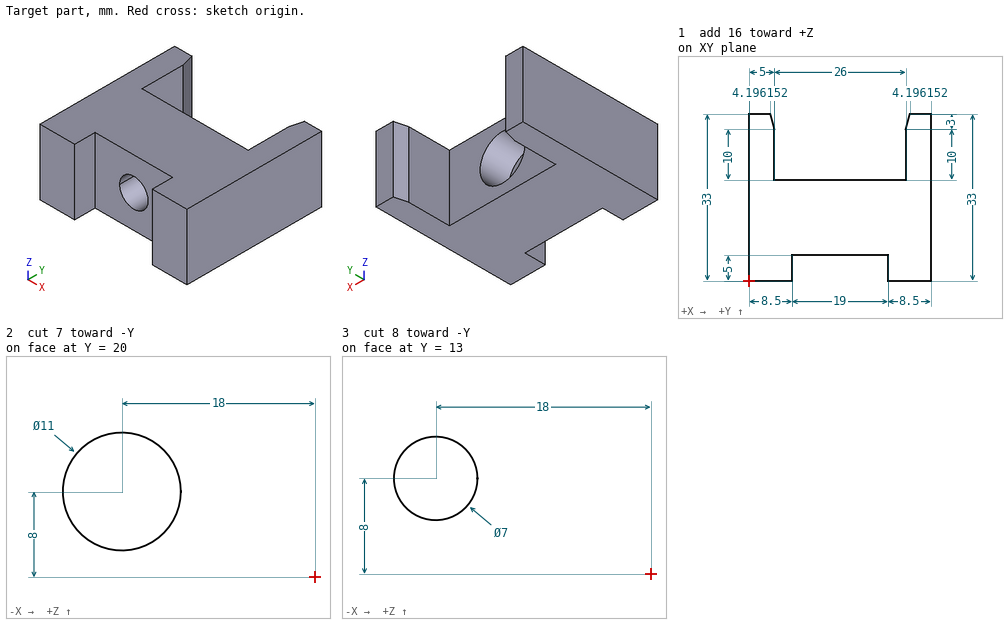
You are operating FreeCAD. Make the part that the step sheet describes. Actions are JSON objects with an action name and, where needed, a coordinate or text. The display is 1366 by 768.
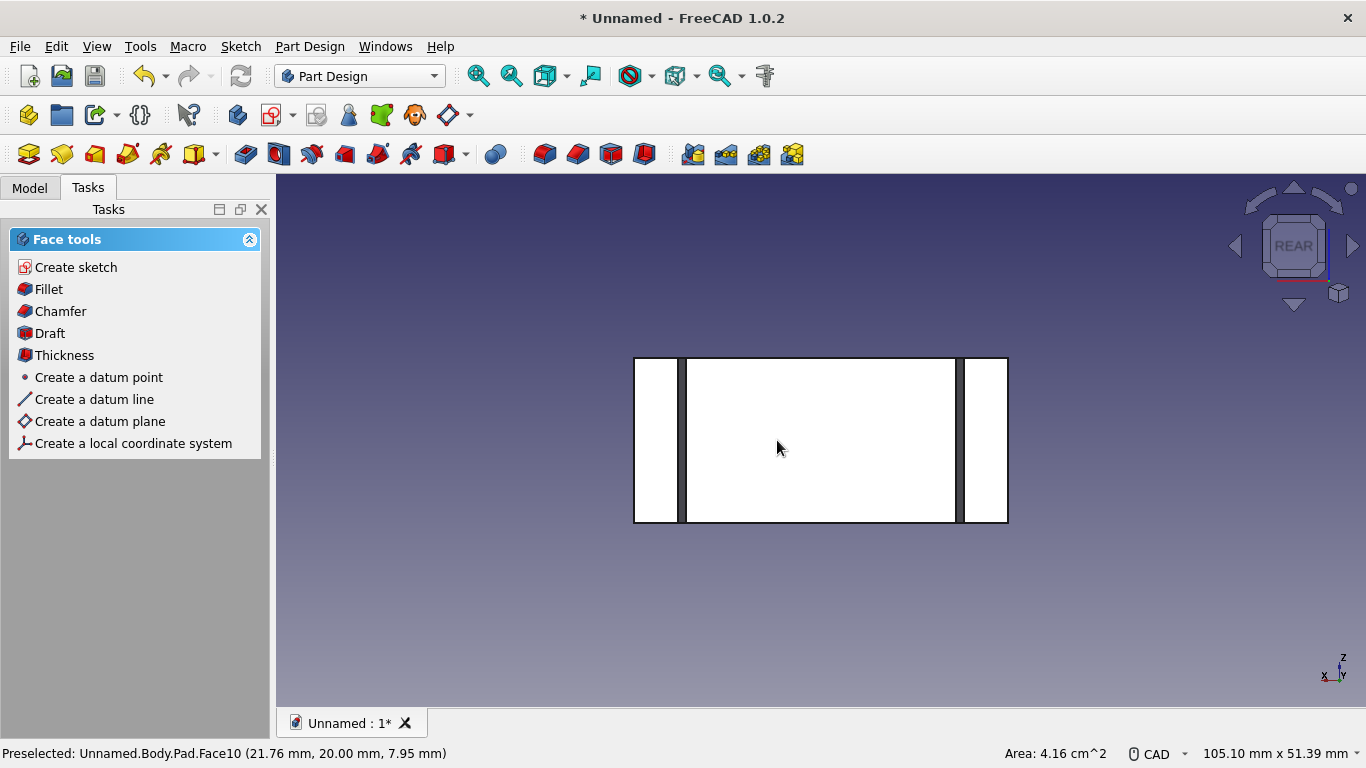
{"action": "left_click", "coordinate": [270, 116]}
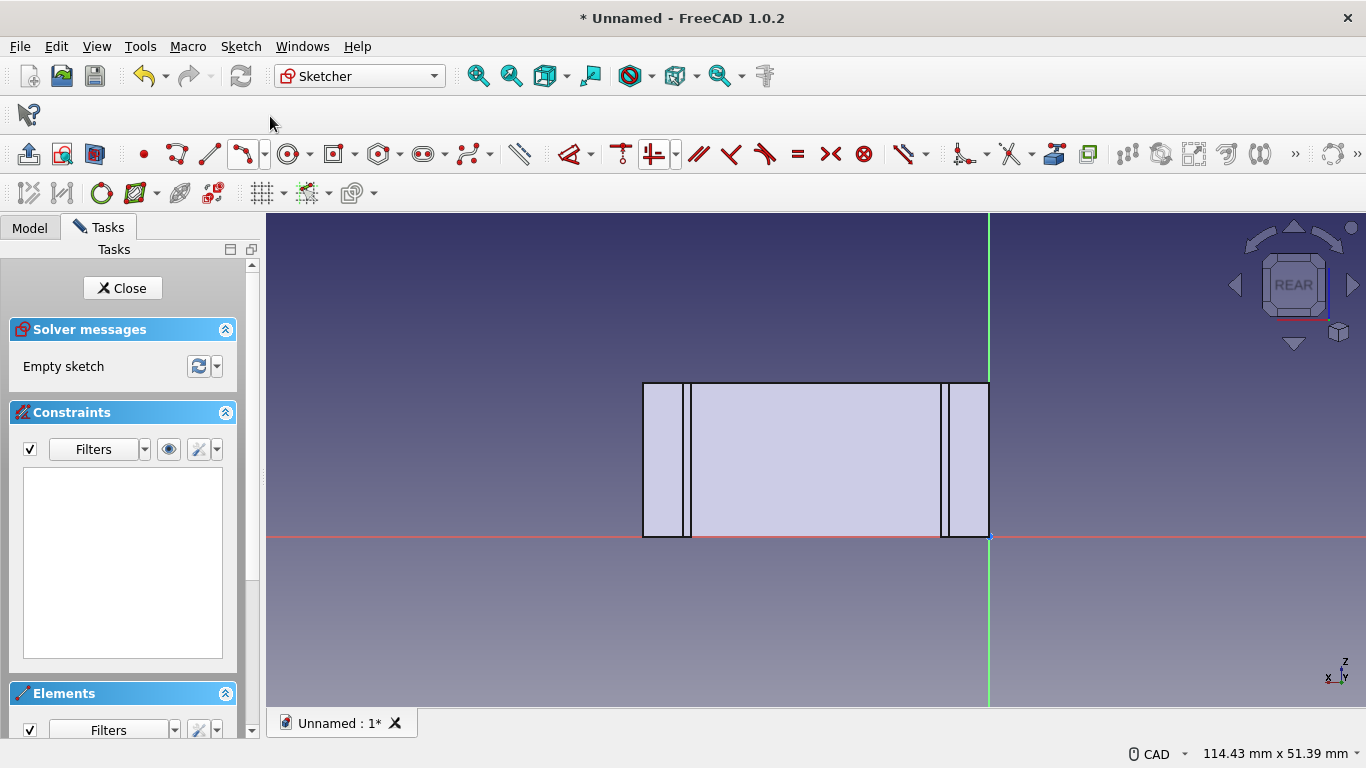
{"action": "left_click", "coordinate": [95, 154]}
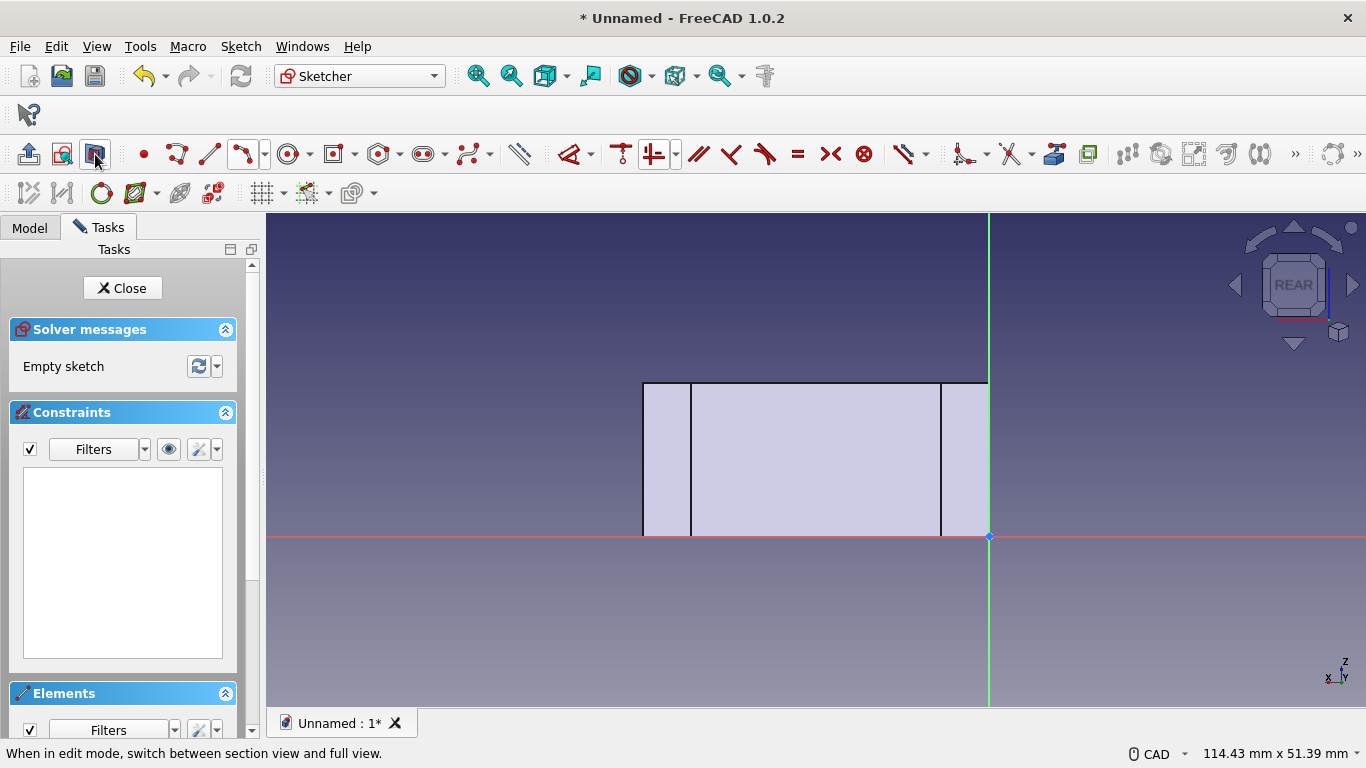
{"action": "scroll", "coordinate": [981, 482], "scroll_direction": "up", "scroll_amount": 4}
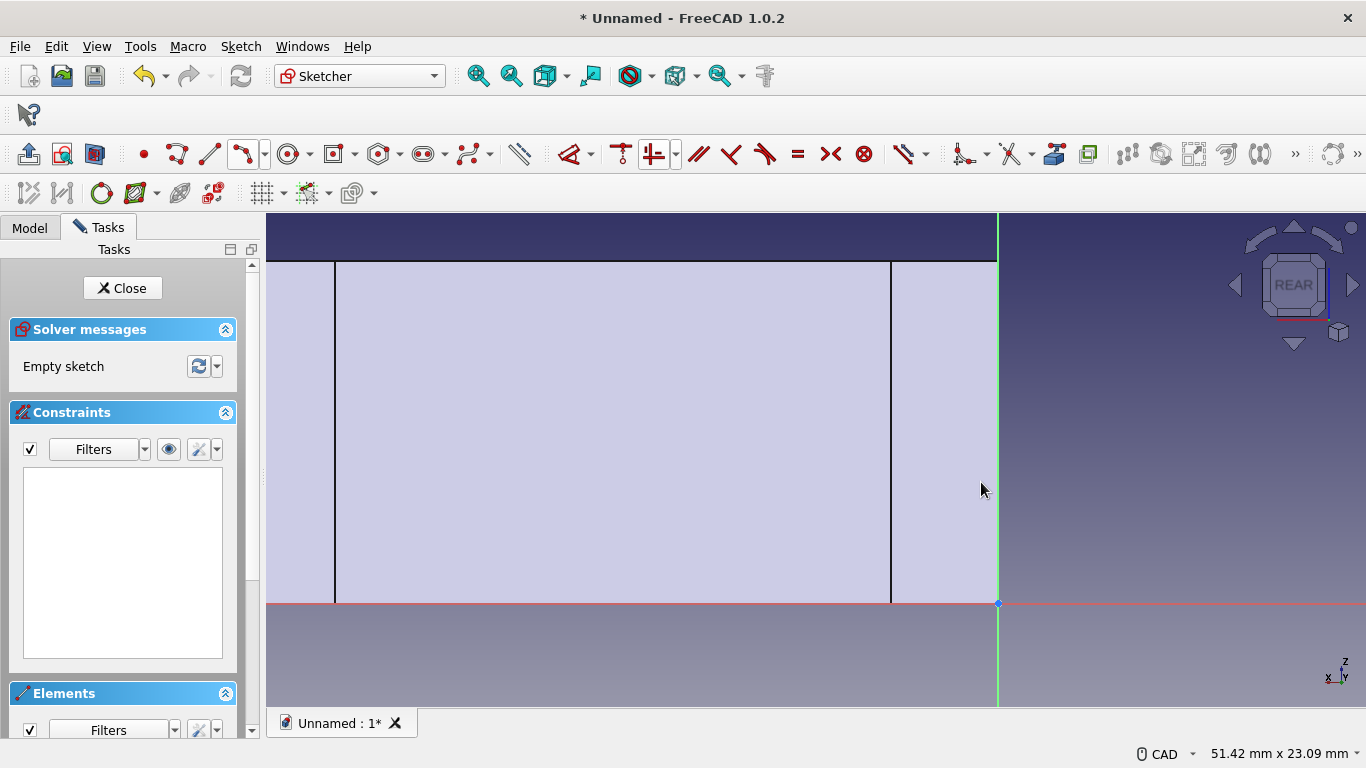
{"action": "left_click", "coordinate": [288, 154]}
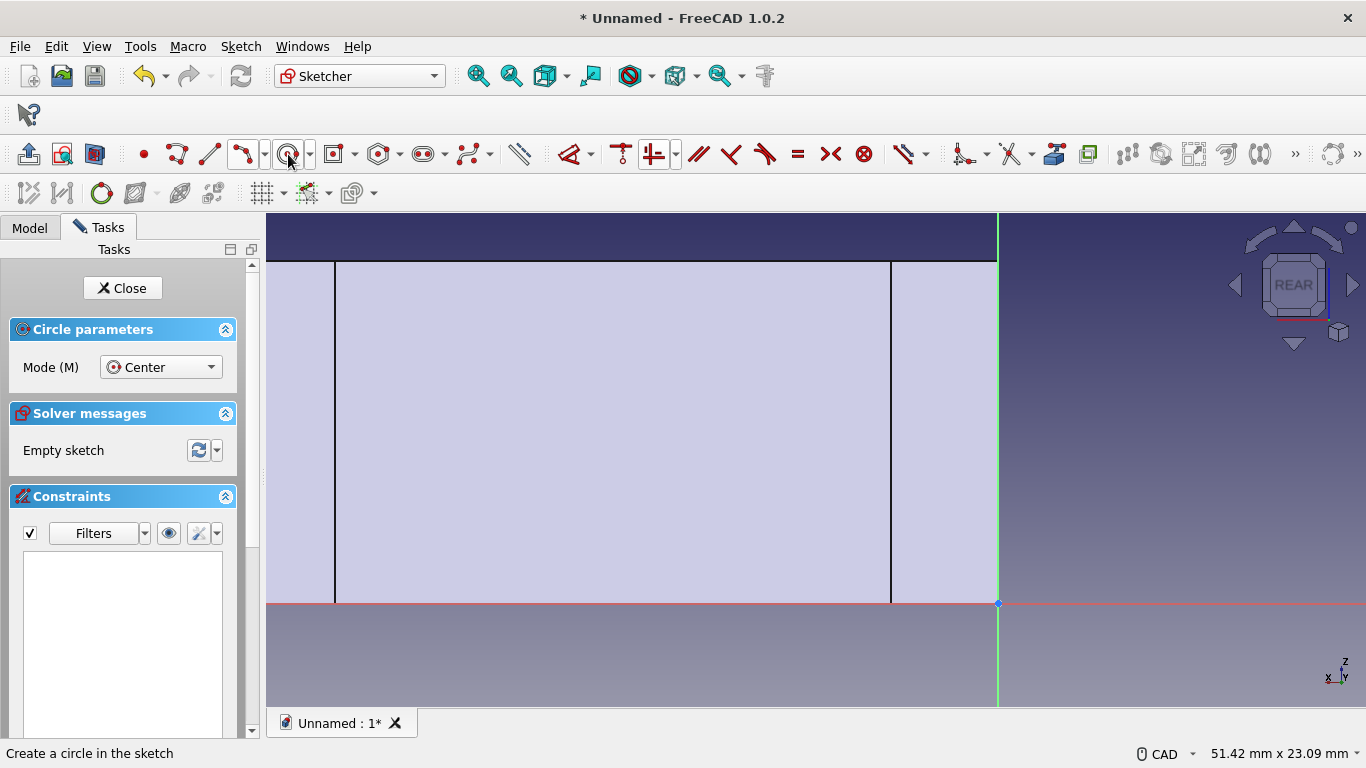
{"action": "left_click", "coordinate": [613, 432]}
{"action": "mouse_move", "coordinate": [696, 349]}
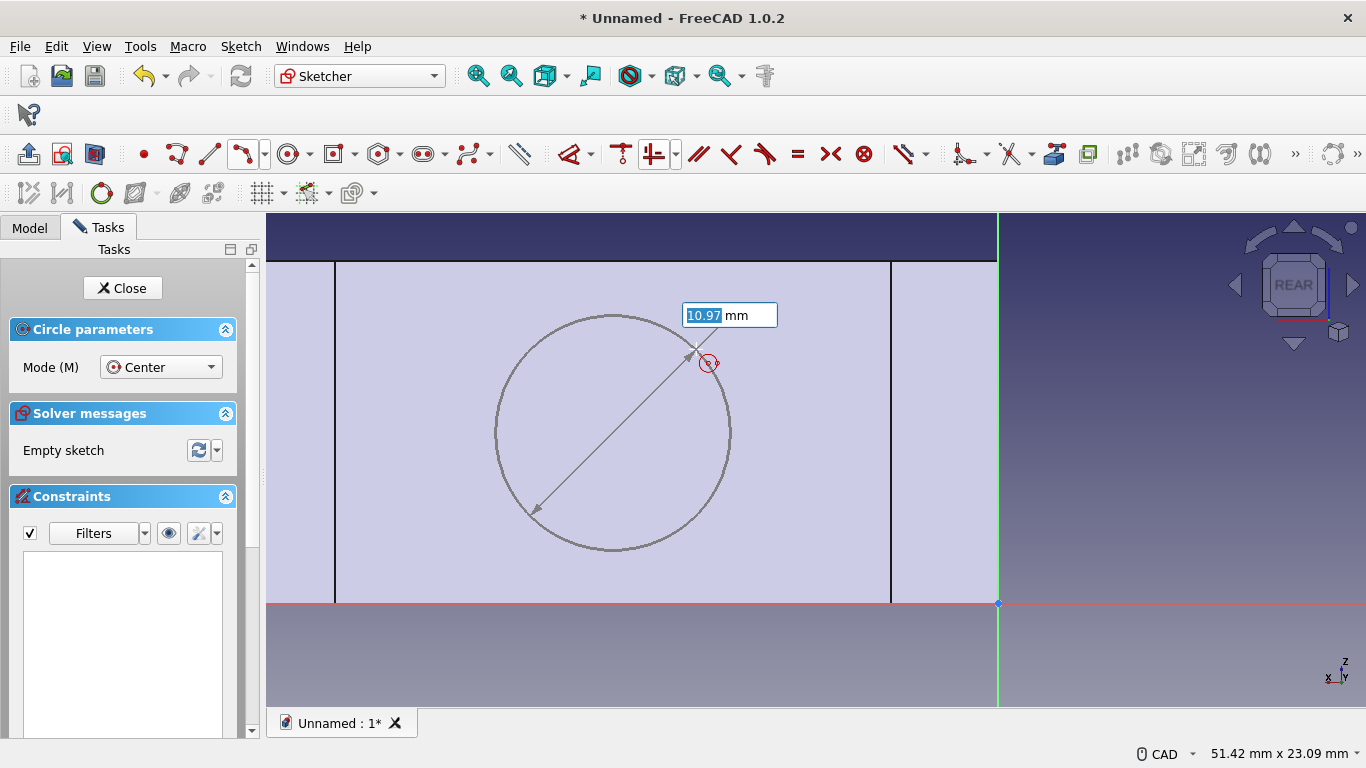
{"action": "type", "text": "11"}
{"action": "key", "text": "Return"}
{"action": "key", "text": "Escape"}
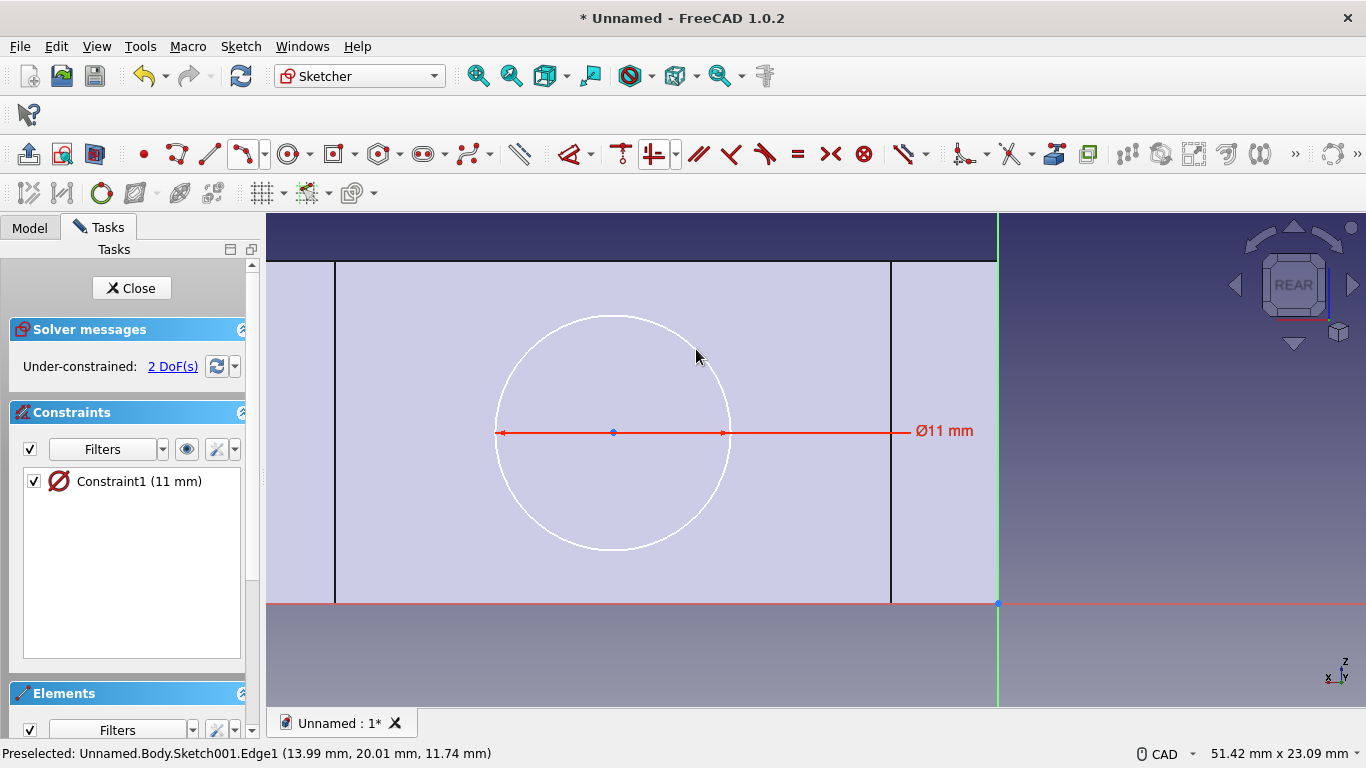
{"action": "left_click", "coordinate": [568, 154]}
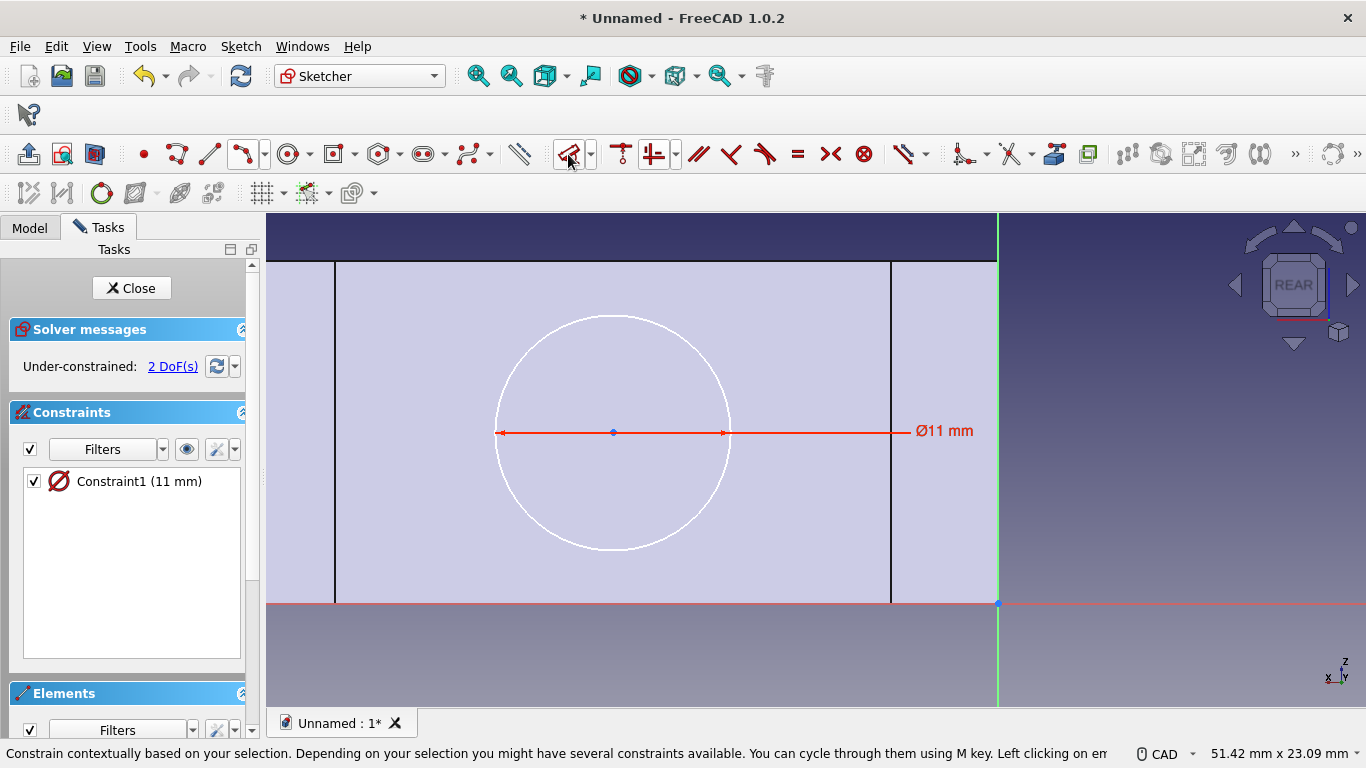
{"action": "left_click", "coordinate": [613, 433]}
{"action": "left_click", "coordinate": [1032, 518]}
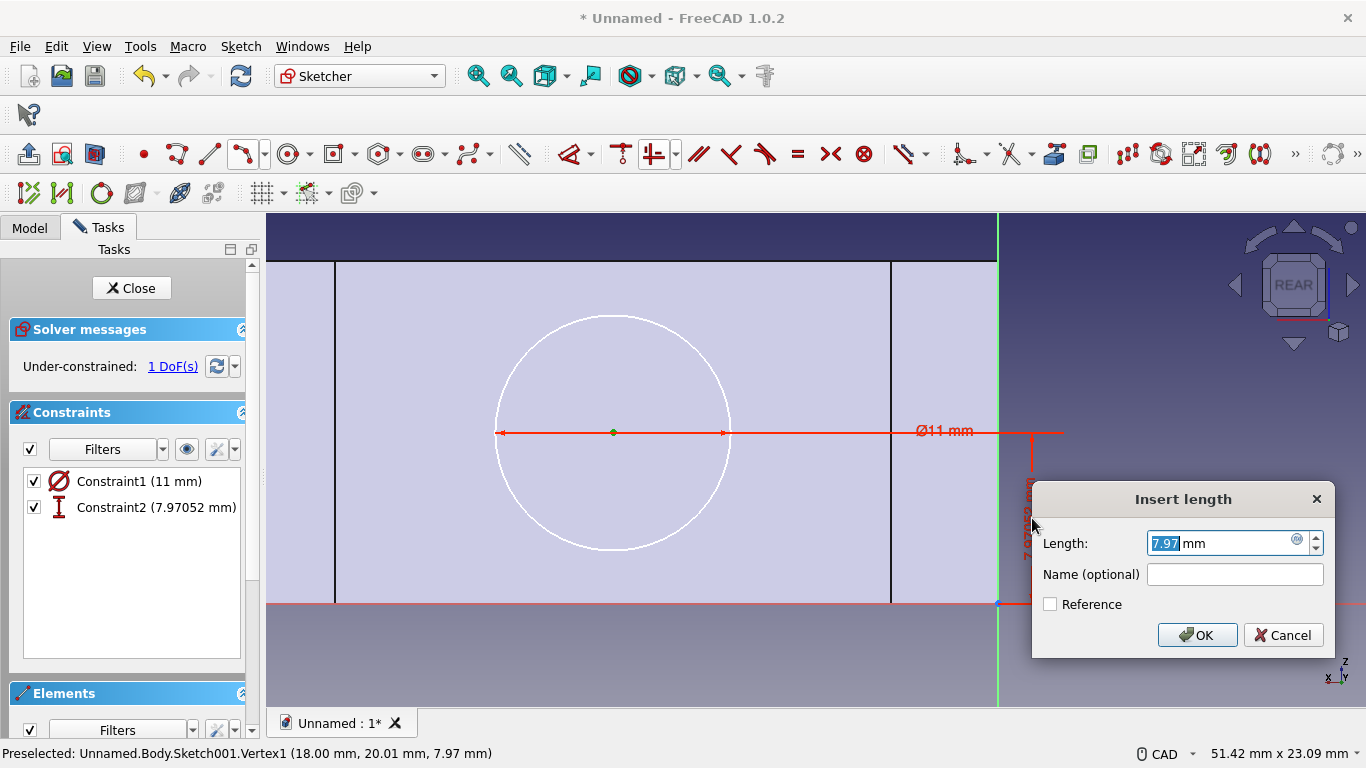
{"action": "type", "text": "8"}
{"action": "key", "text": "Return"}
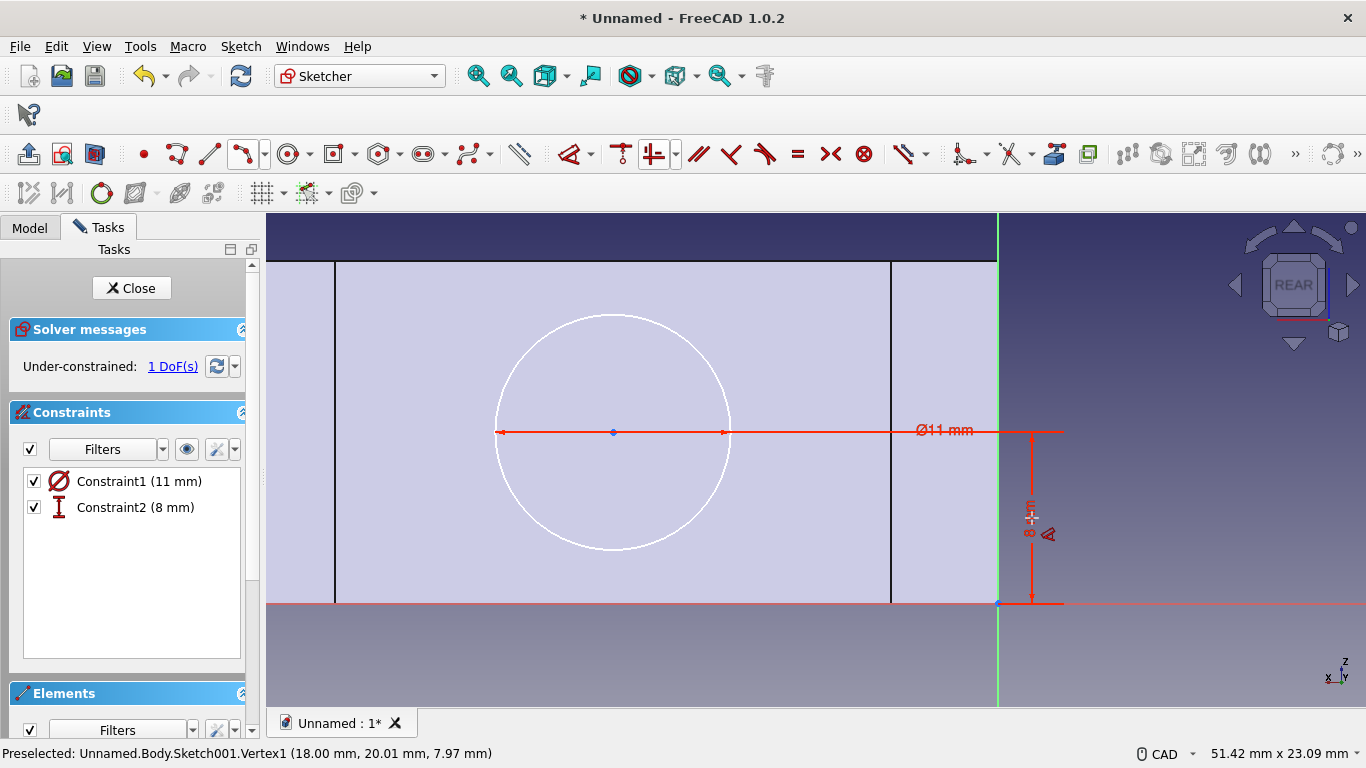
{"action": "left_click", "coordinate": [613, 432]}
{"action": "left_click", "coordinate": [806, 638]}